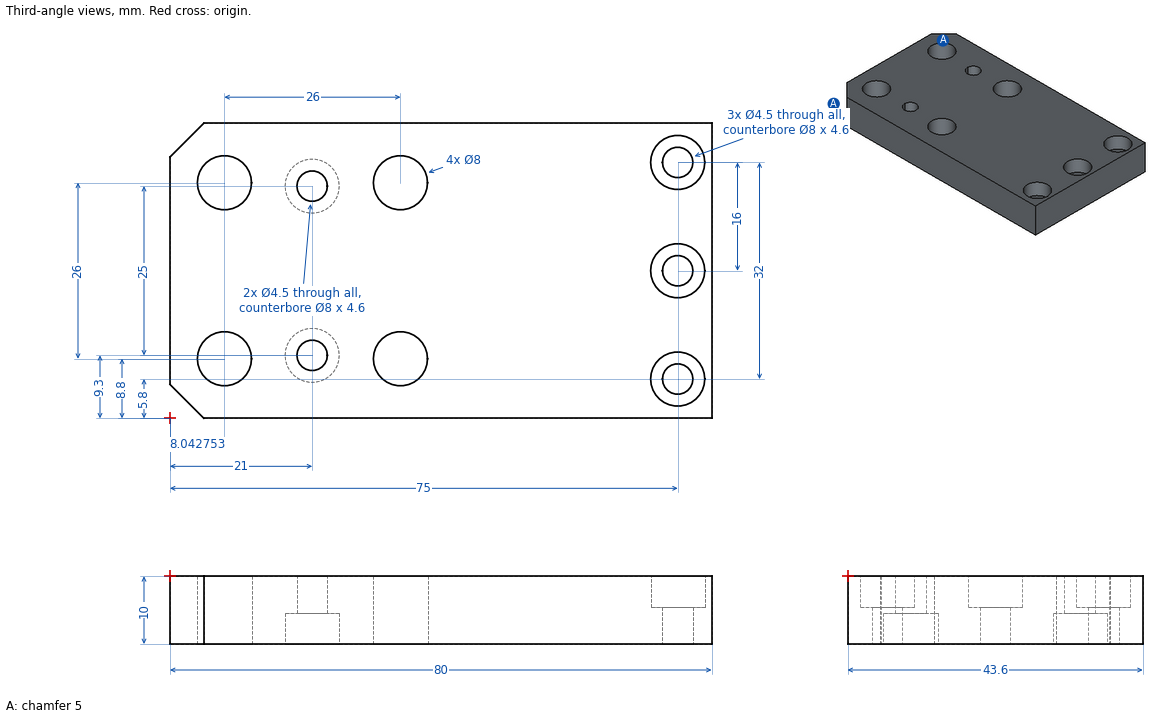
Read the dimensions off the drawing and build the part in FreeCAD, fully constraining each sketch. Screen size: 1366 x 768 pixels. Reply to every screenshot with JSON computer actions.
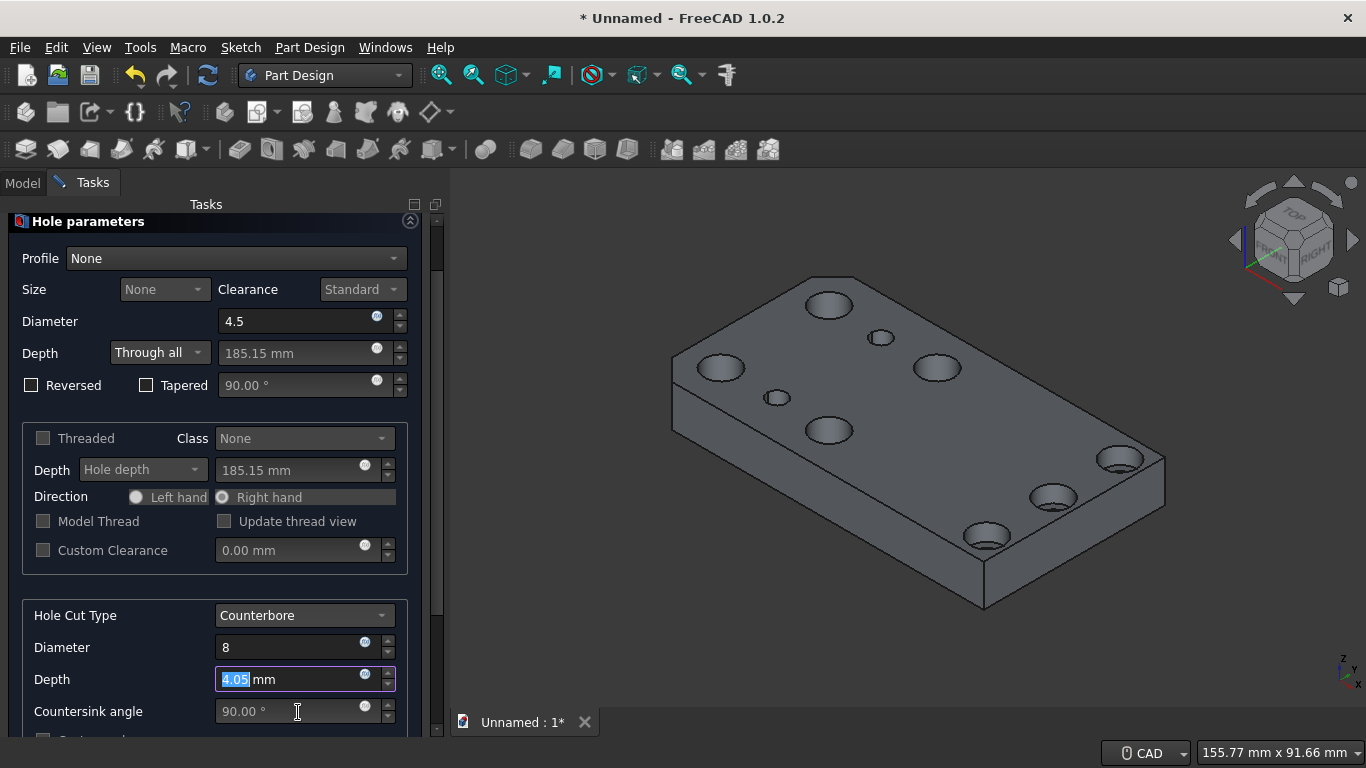
{"action": "type", "text": "4.6"}
{"action": "key", "text": "Tab"}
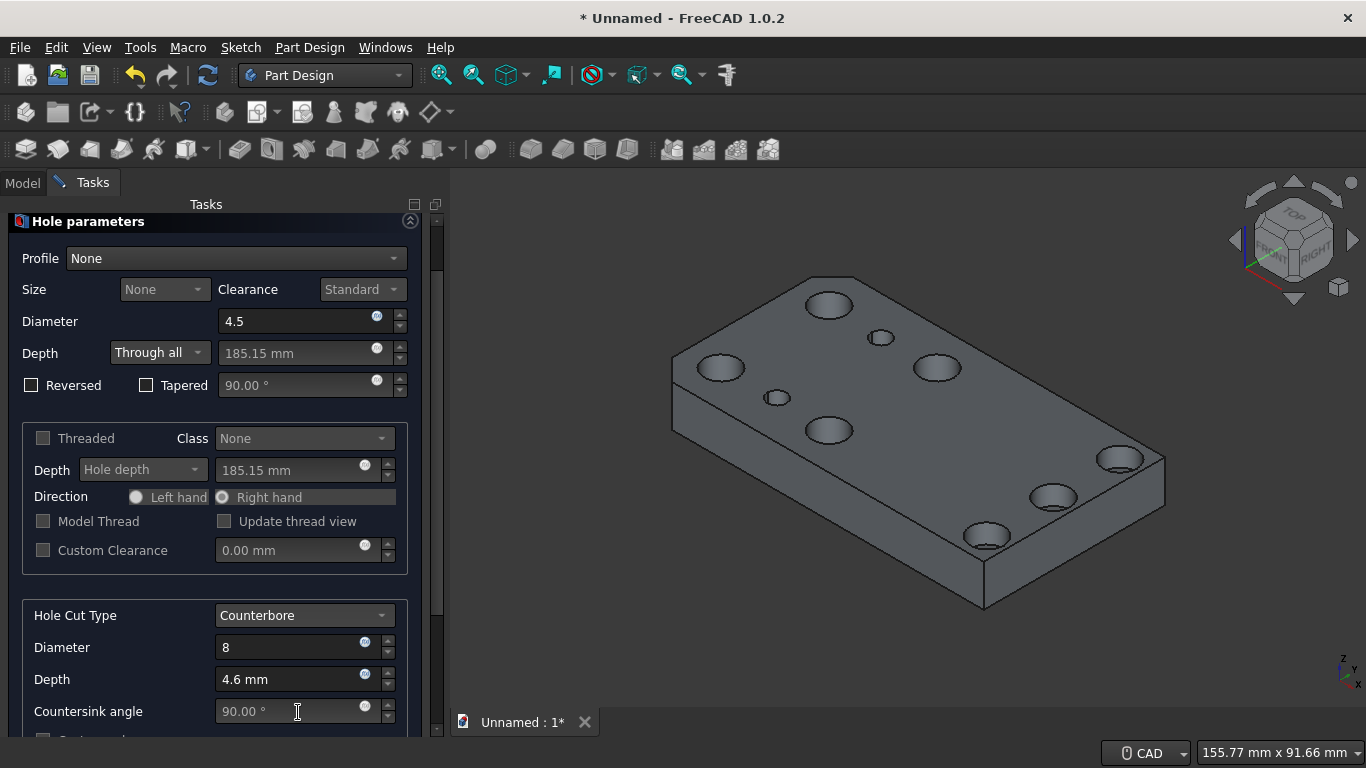
{"action": "scroll", "coordinate": [437, 475], "scroll_direction": "up", "scroll_amount": 2}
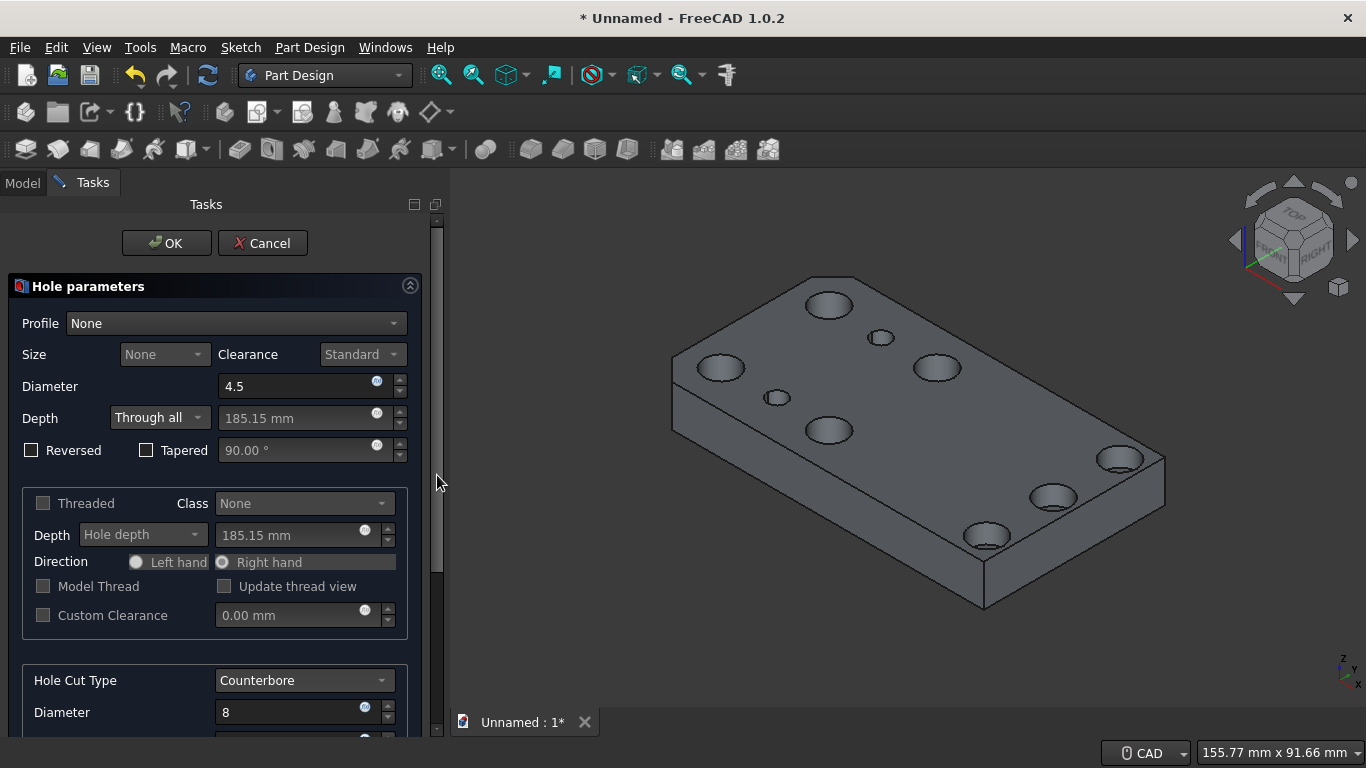
{"action": "left_click", "coordinate": [167, 243]}